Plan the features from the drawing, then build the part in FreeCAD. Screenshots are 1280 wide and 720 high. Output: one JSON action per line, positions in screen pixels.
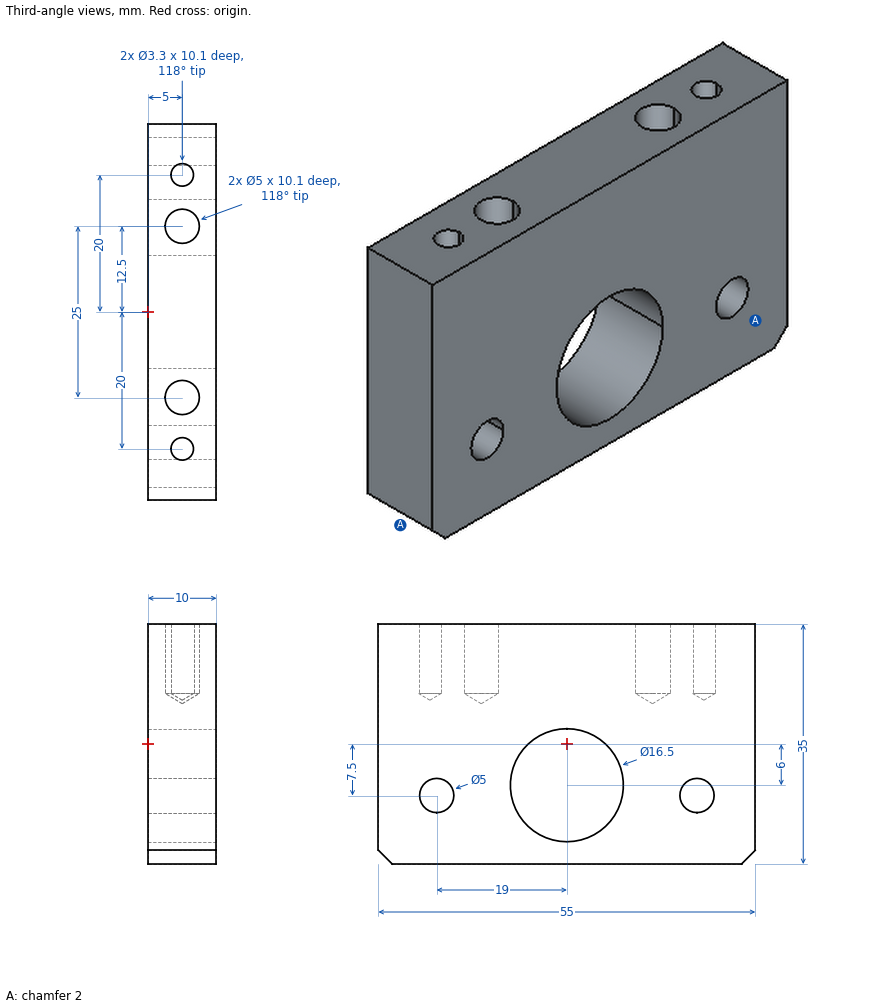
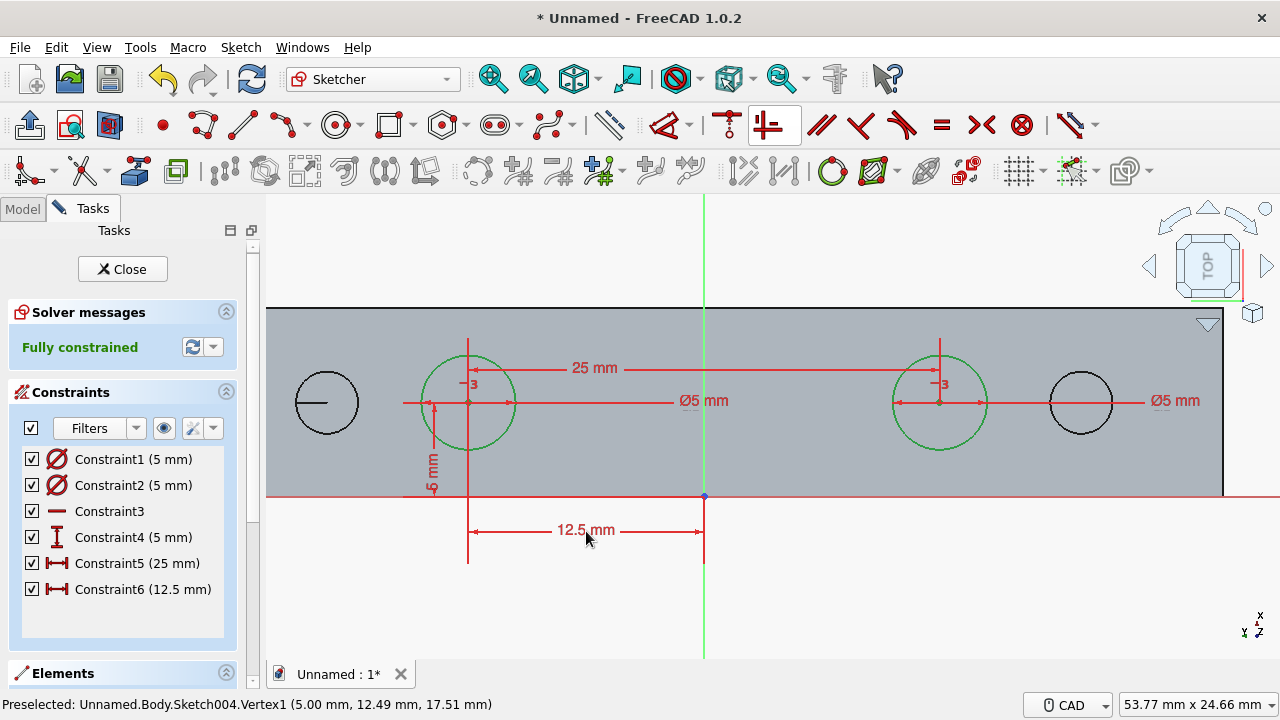
{"action": "left_click", "coordinate": [123, 269]}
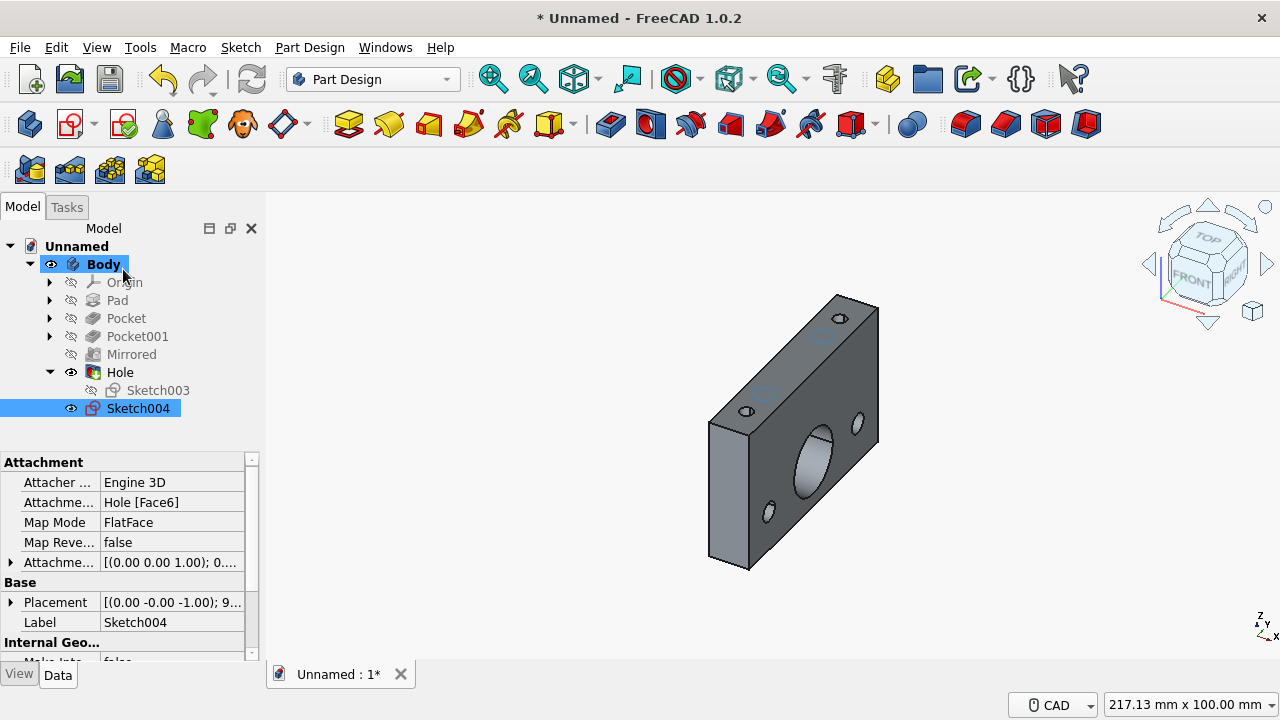
{"action": "left_click", "coordinate": [652, 124]}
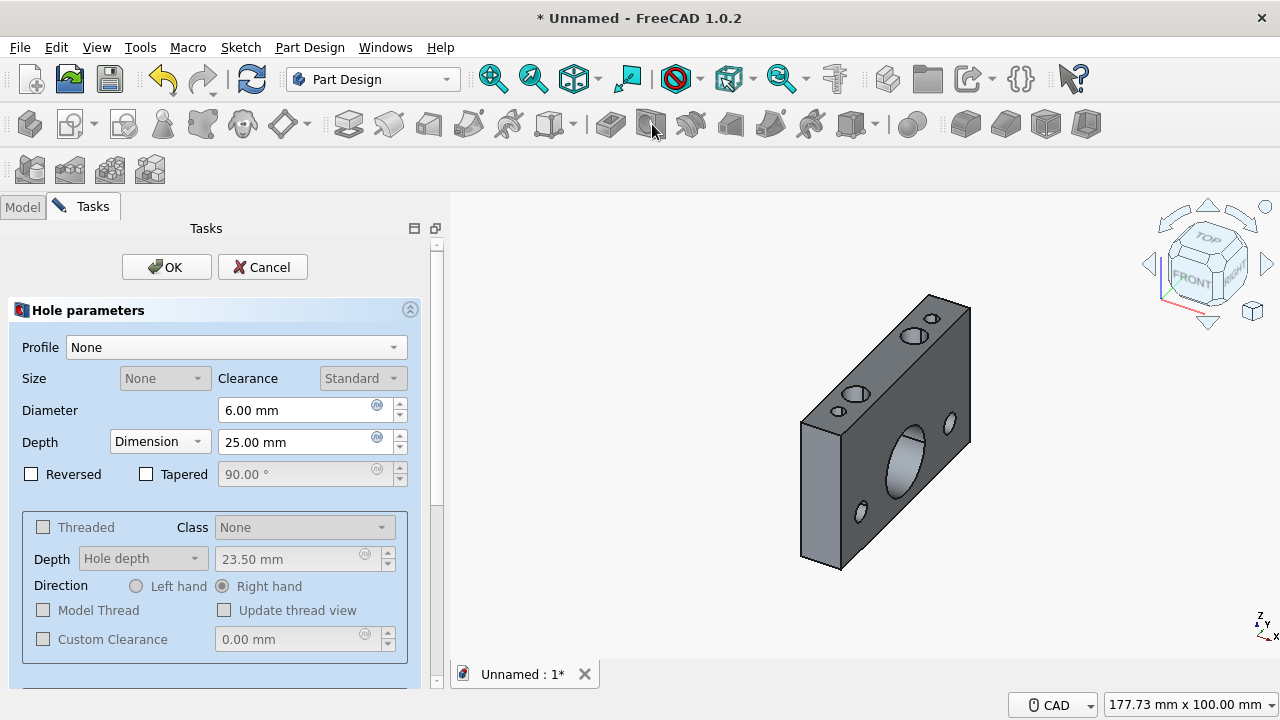
{"action": "triple_click", "coordinate": [305, 410]}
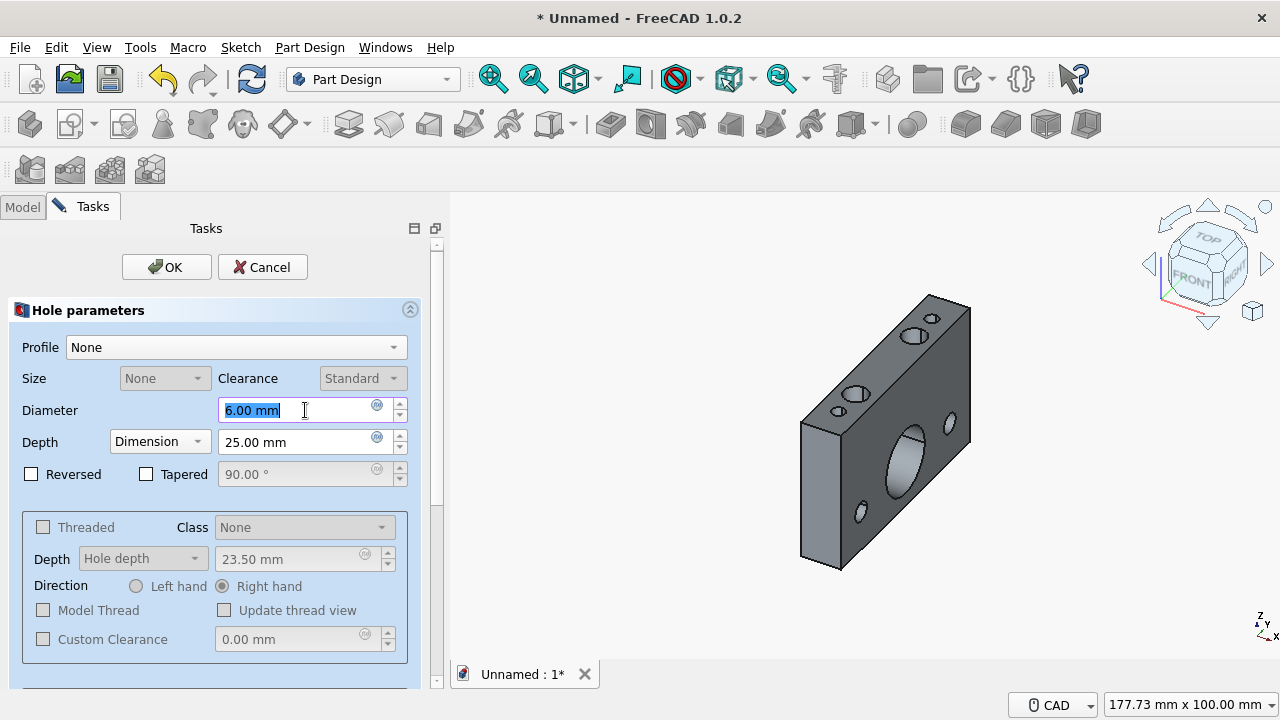
{"action": "type", "text": "5"}
{"action": "key", "text": "Tab"}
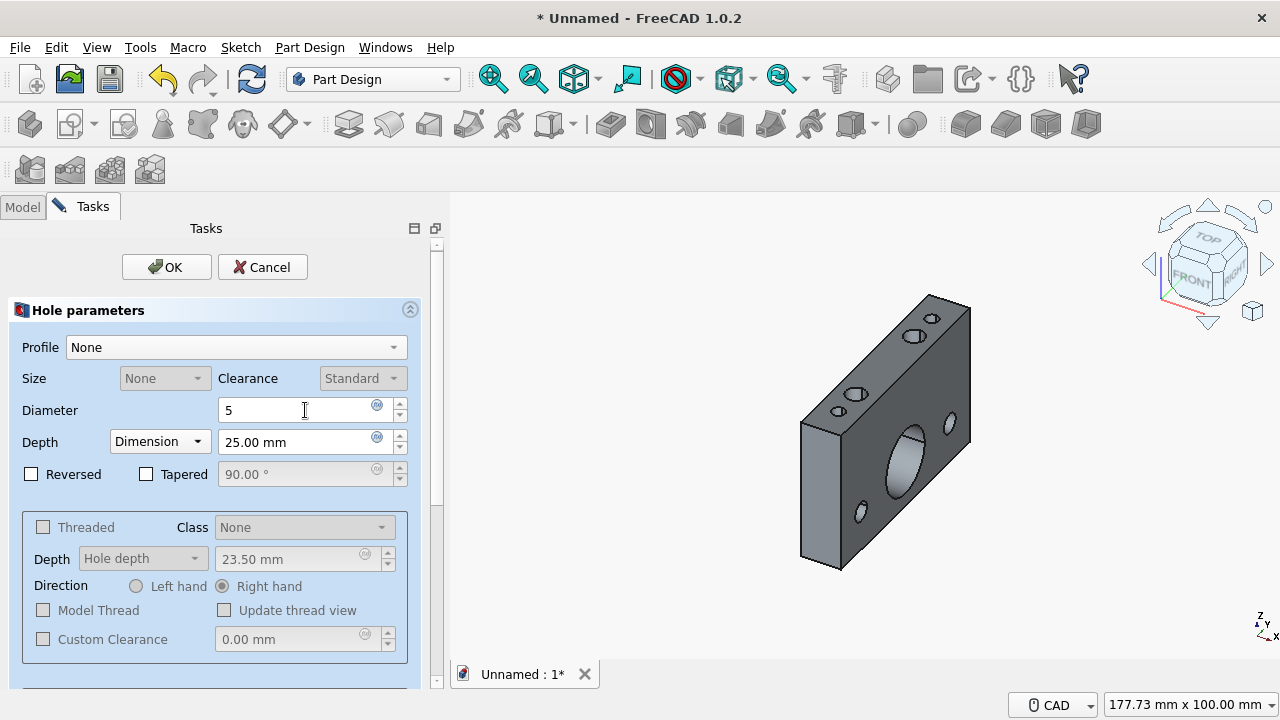
{"action": "triple_click", "coordinate": [305, 442]}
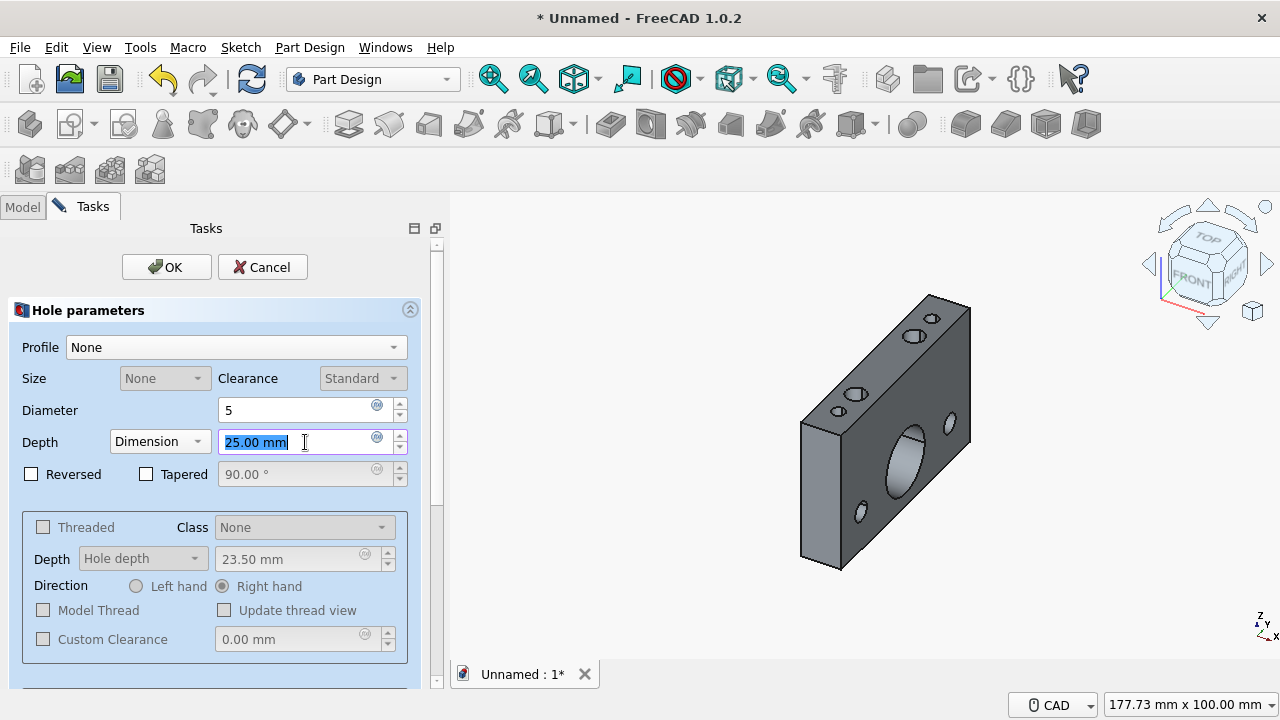
{"action": "type", "text": "10.1"}
{"action": "key", "text": "Tab"}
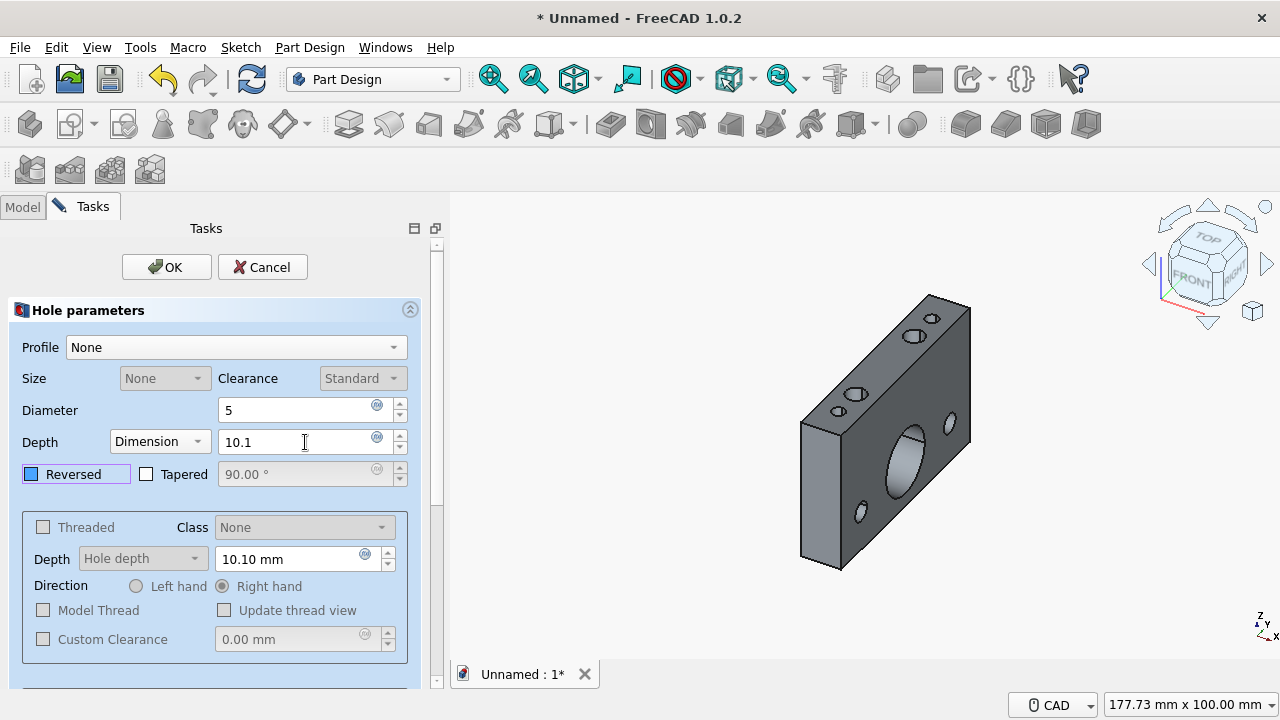
{"action": "left_click", "coordinate": [167, 267]}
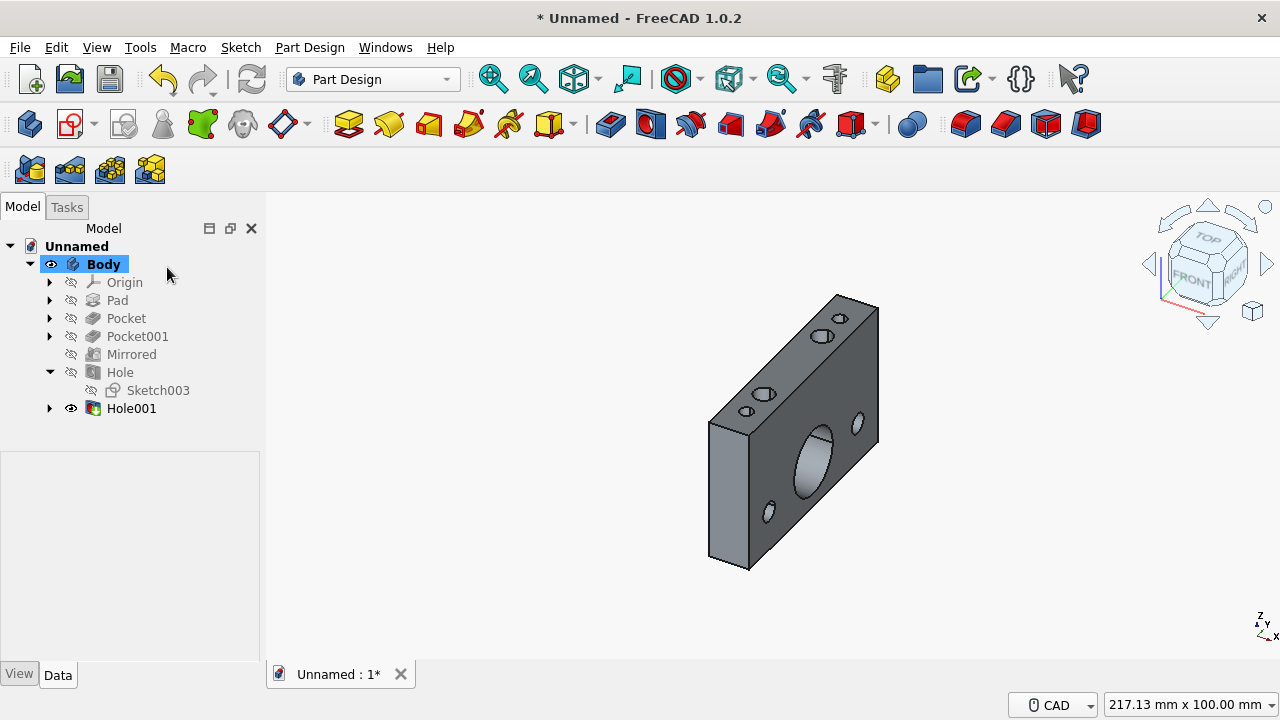
{"action": "key", "text": "0"}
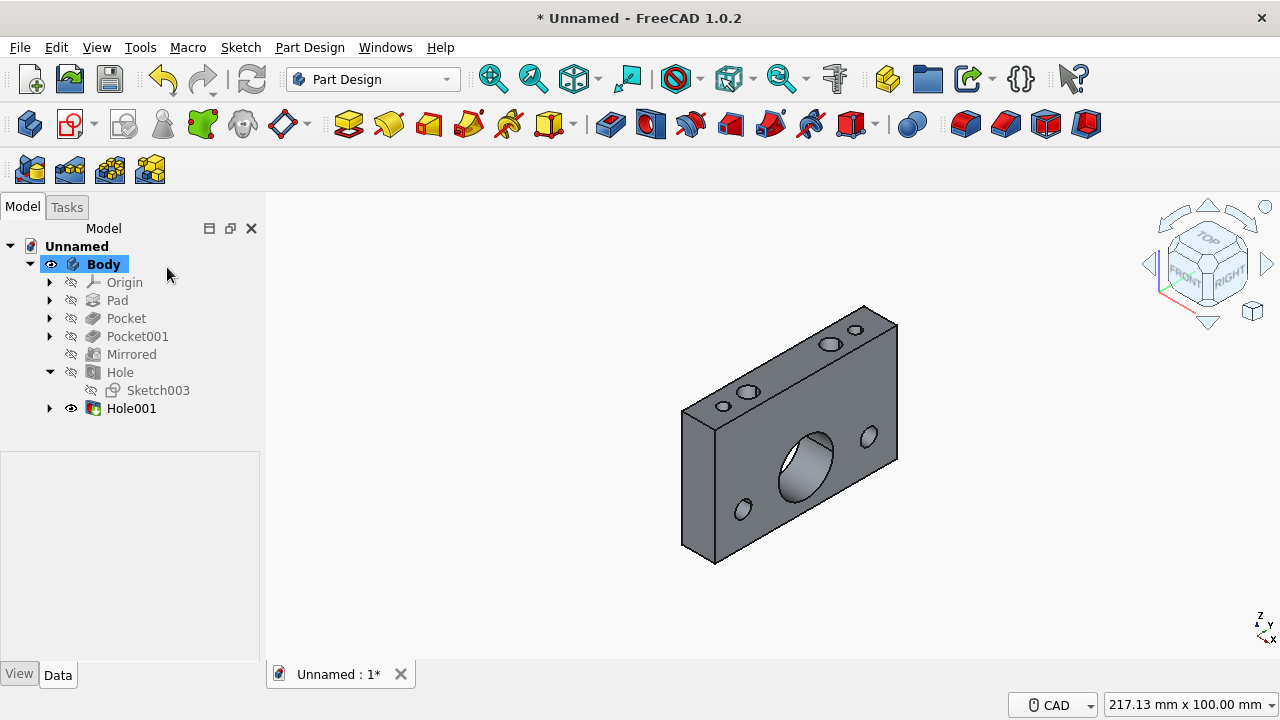
{"action": "key", "text": "2"}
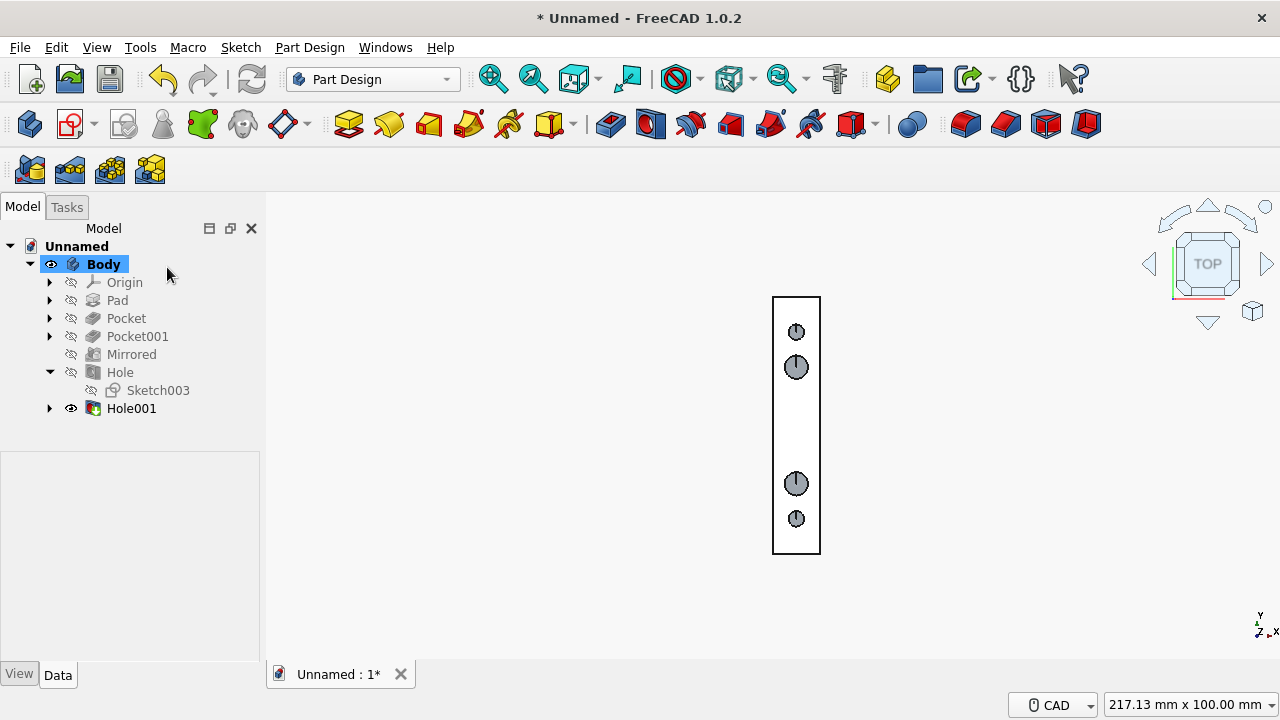
{"action": "key", "text": "1"}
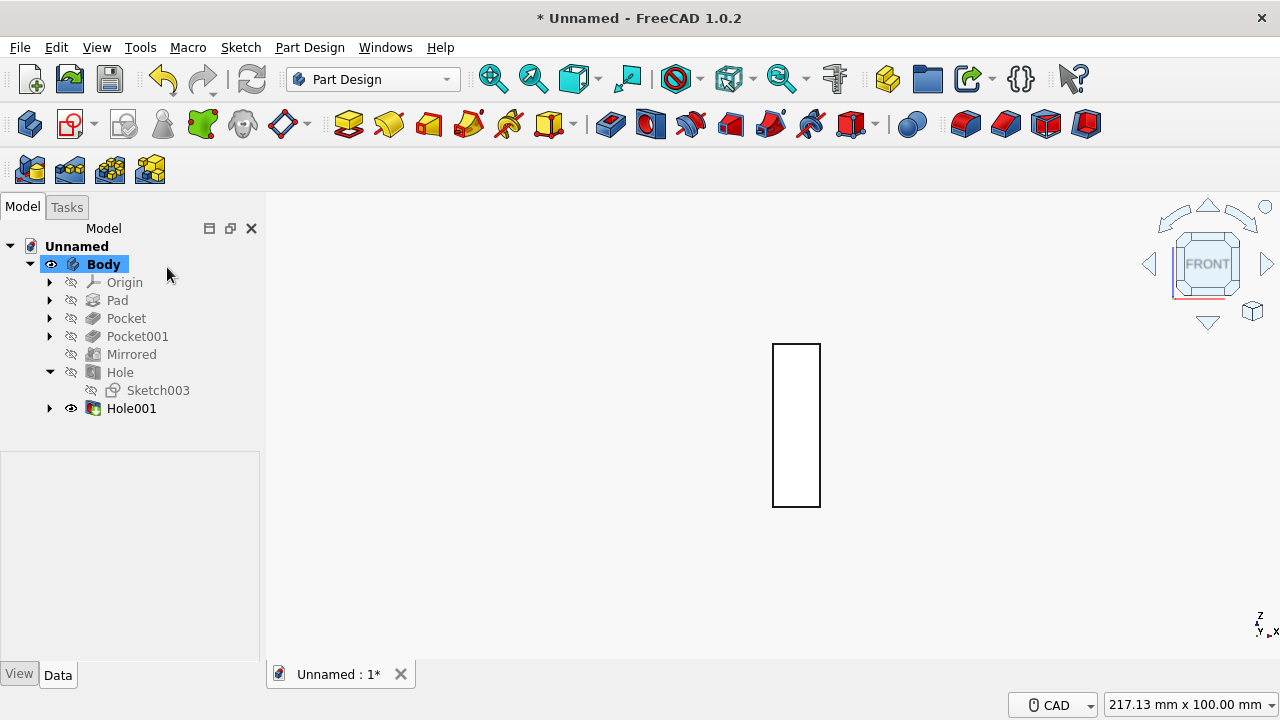
{"action": "left_click", "coordinate": [494, 80]}